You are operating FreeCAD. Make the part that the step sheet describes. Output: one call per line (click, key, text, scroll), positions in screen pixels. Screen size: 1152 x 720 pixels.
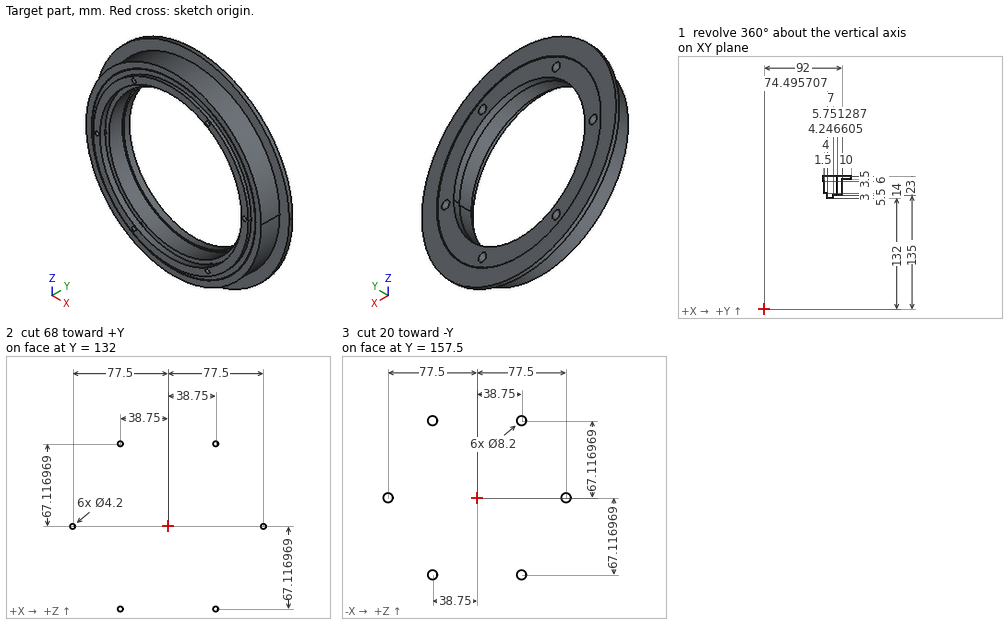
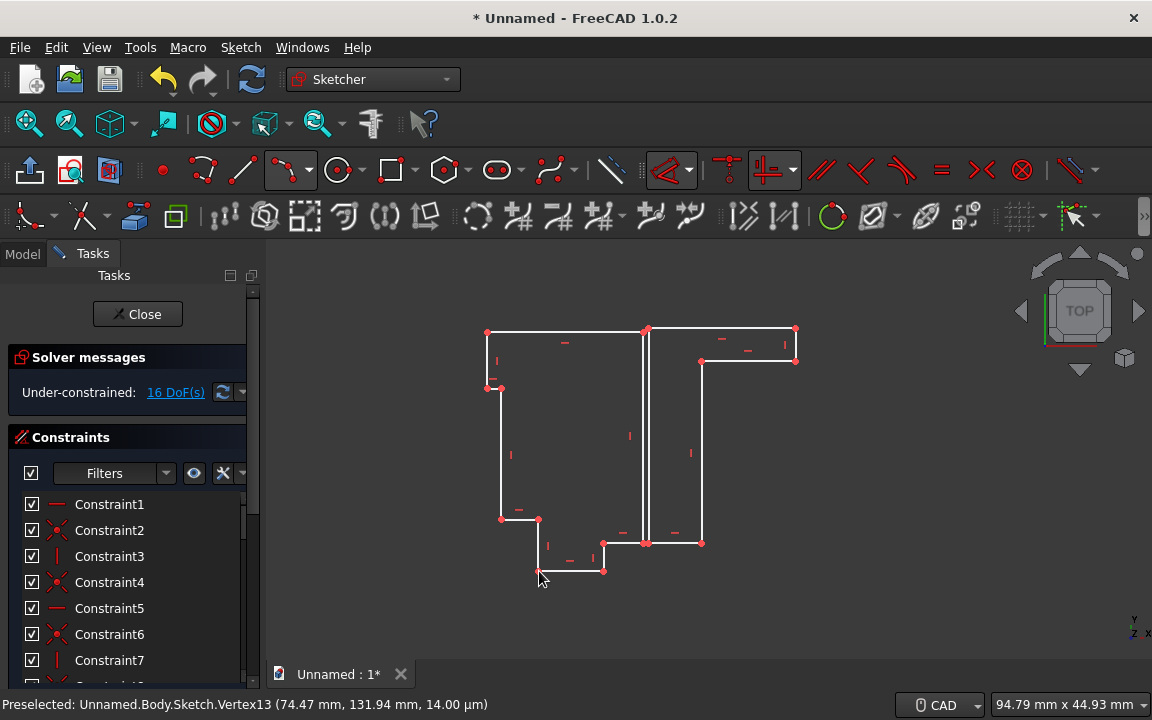
click(666, 170)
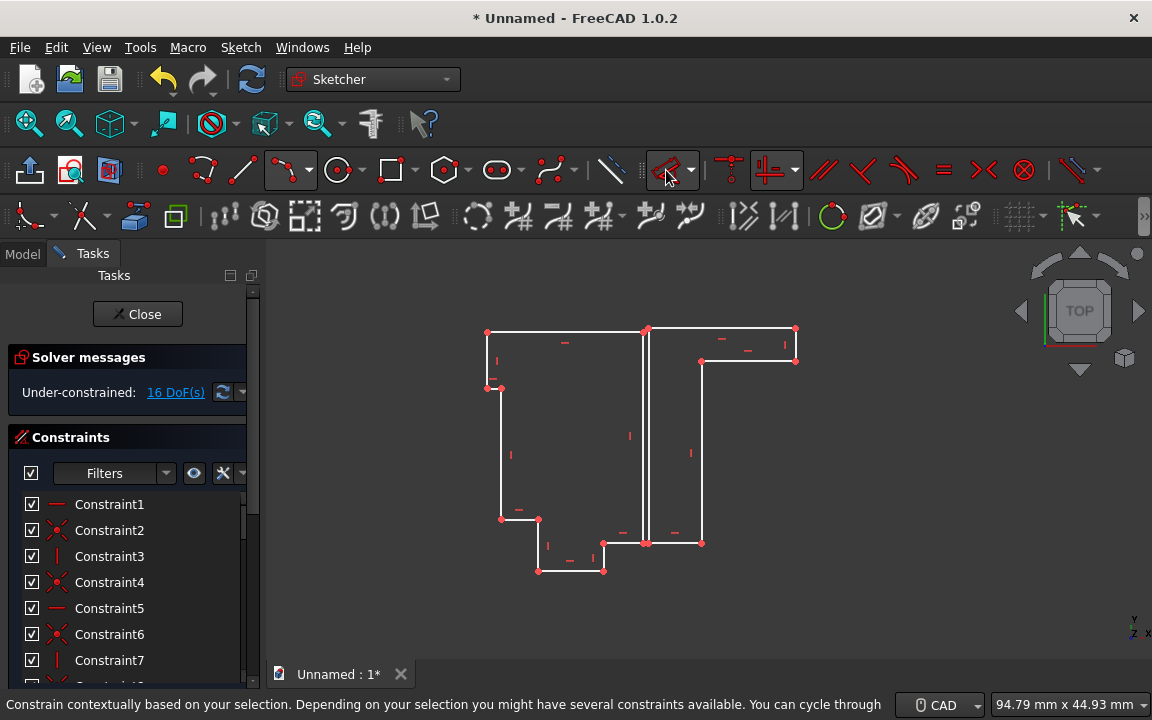
click(558, 571)
click(571, 605)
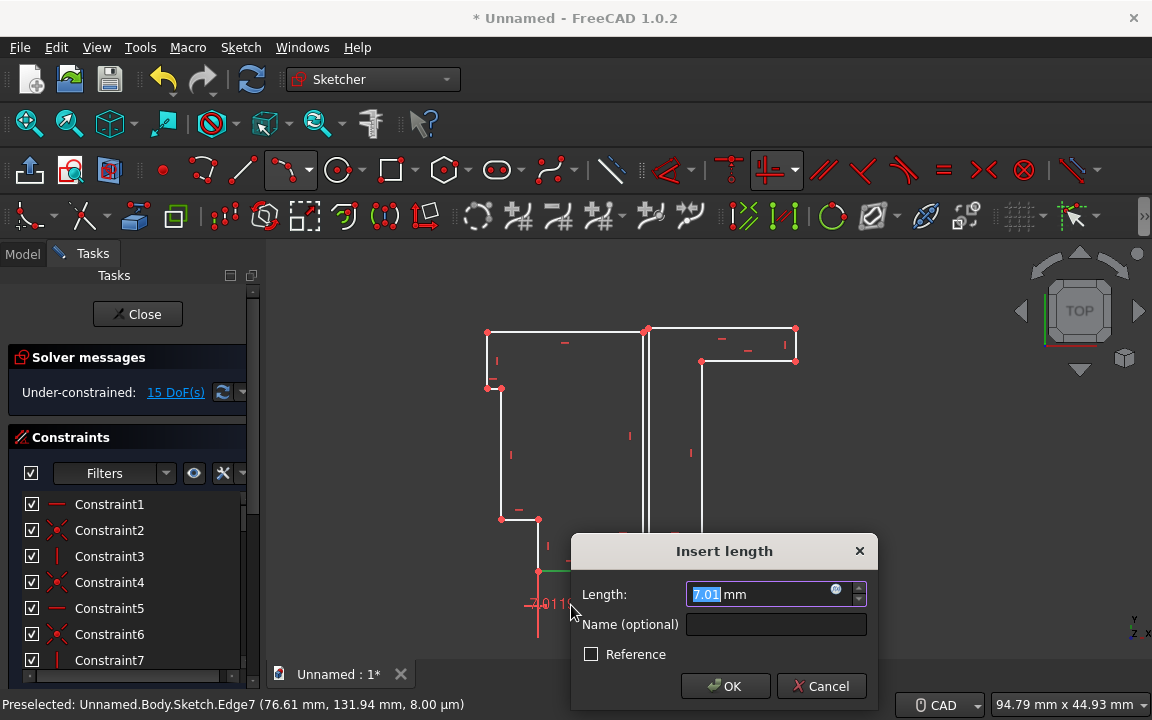
text(7)
key(Return)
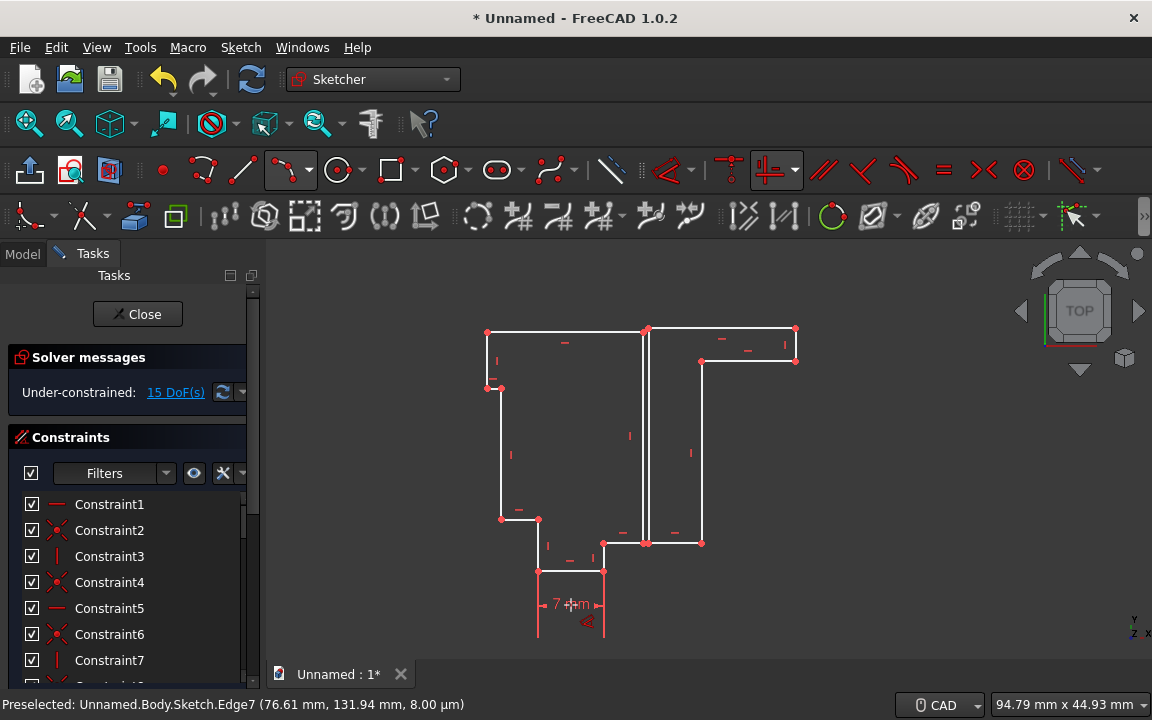
scroll(604, 560, up, 2)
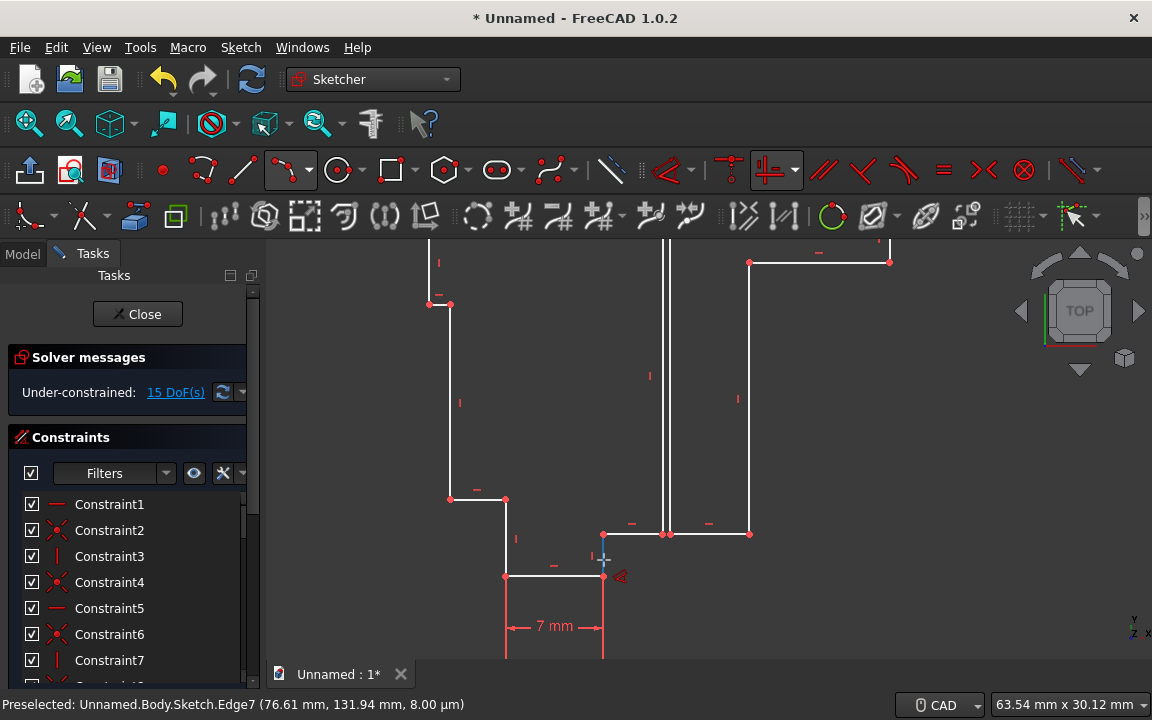
click(603, 559)
click(569, 555)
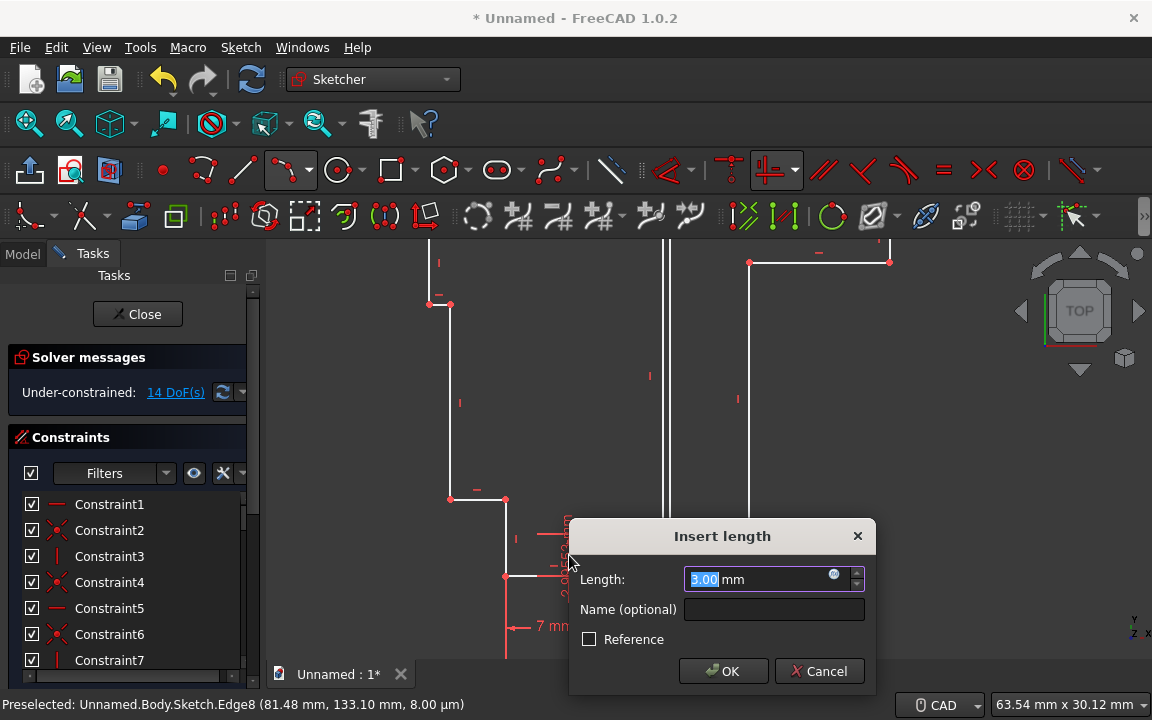
text(3)
key(Return)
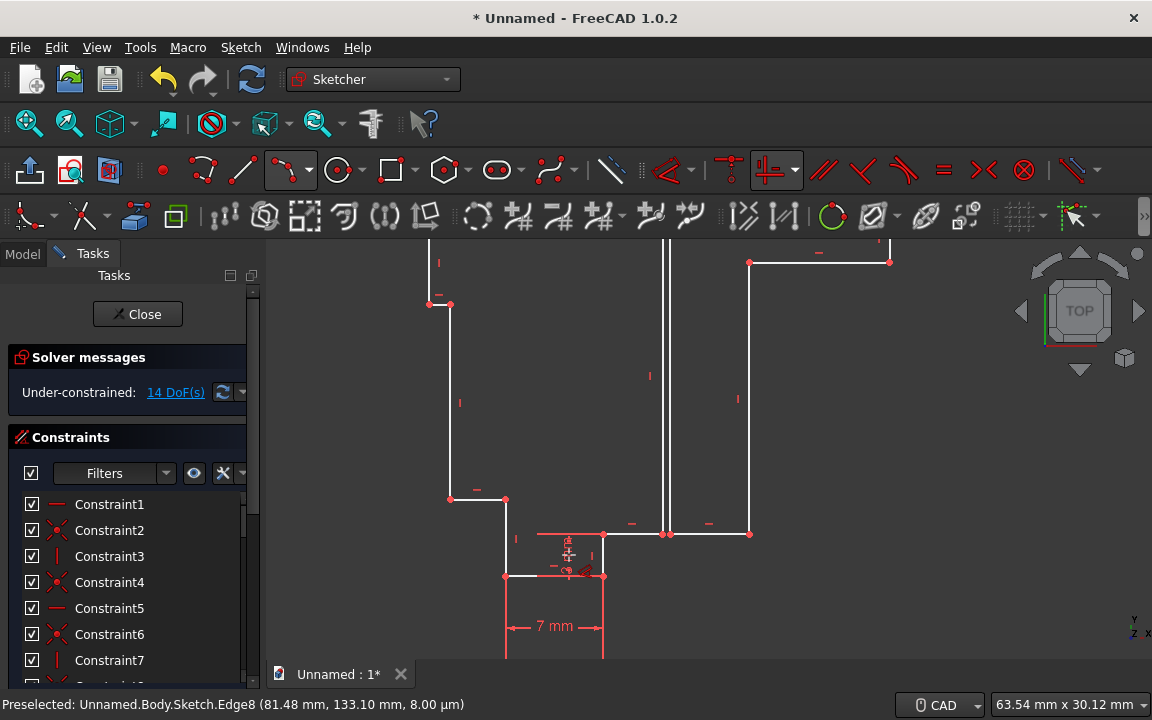
click(429, 279)
click(395, 286)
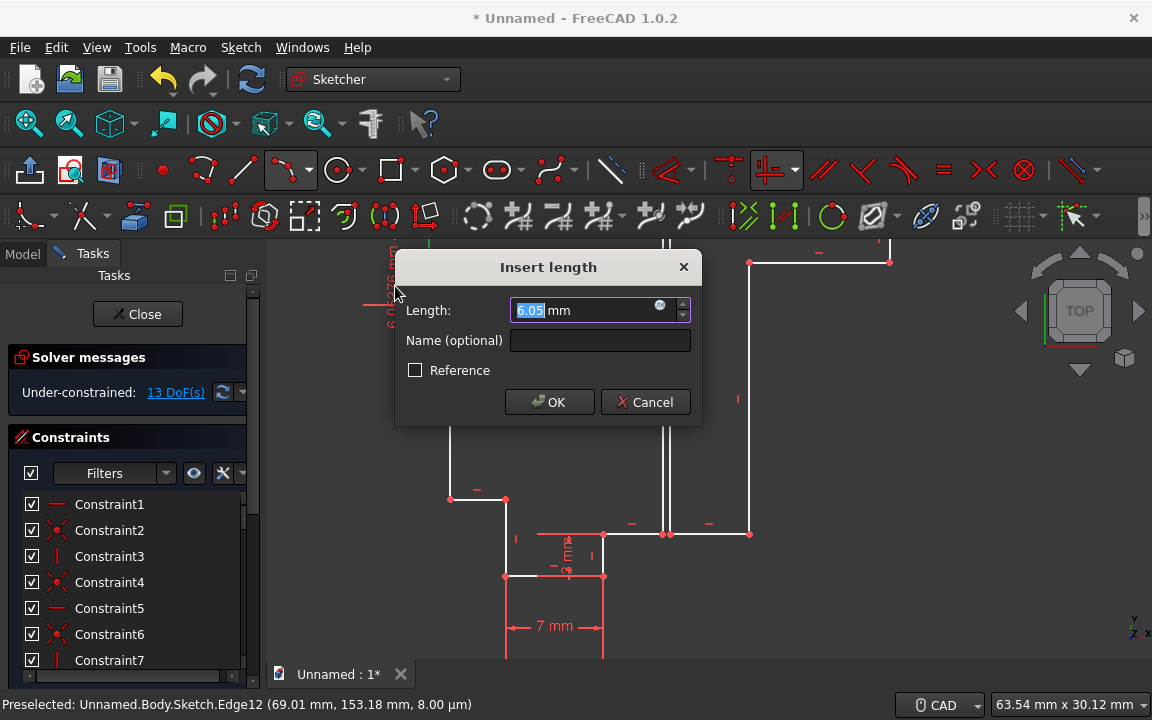
text(6)
key(Return)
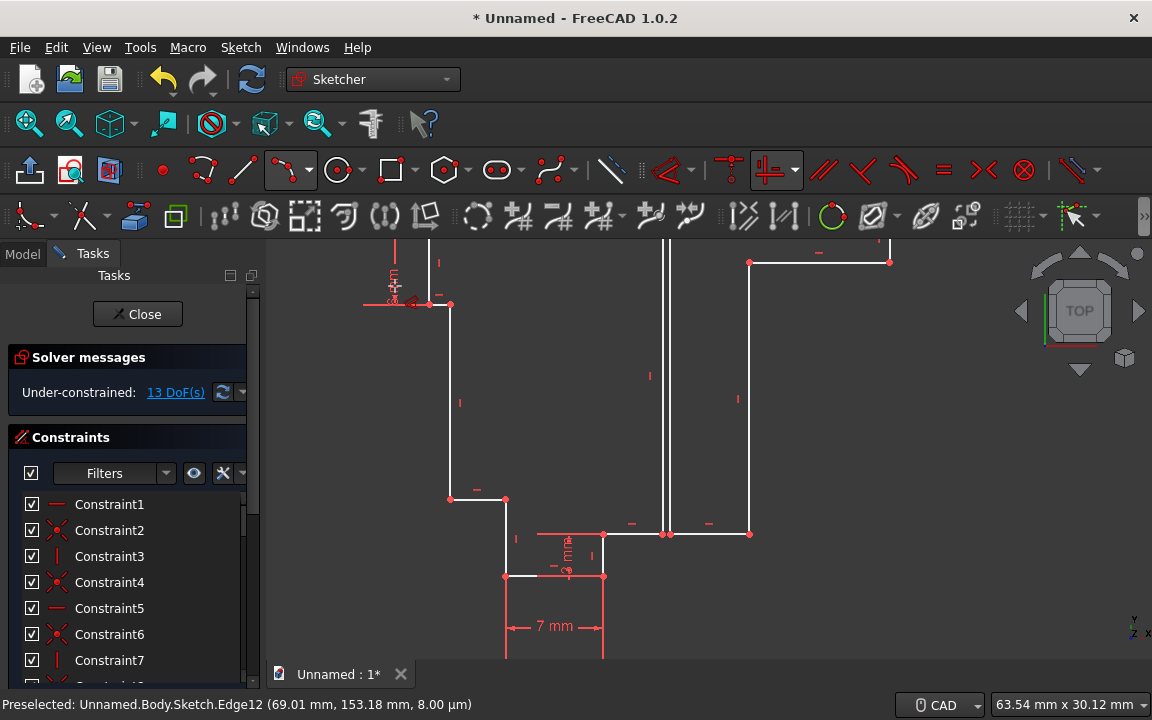
click(467, 500)
click(478, 534)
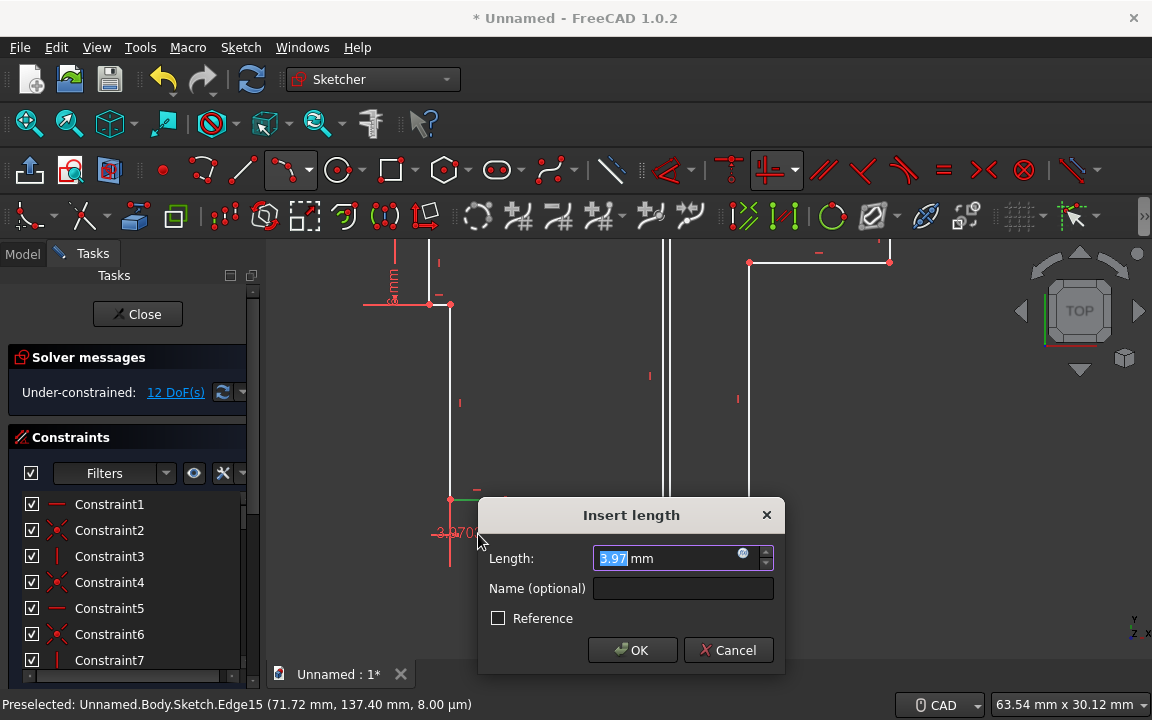
text(4)
key(Return)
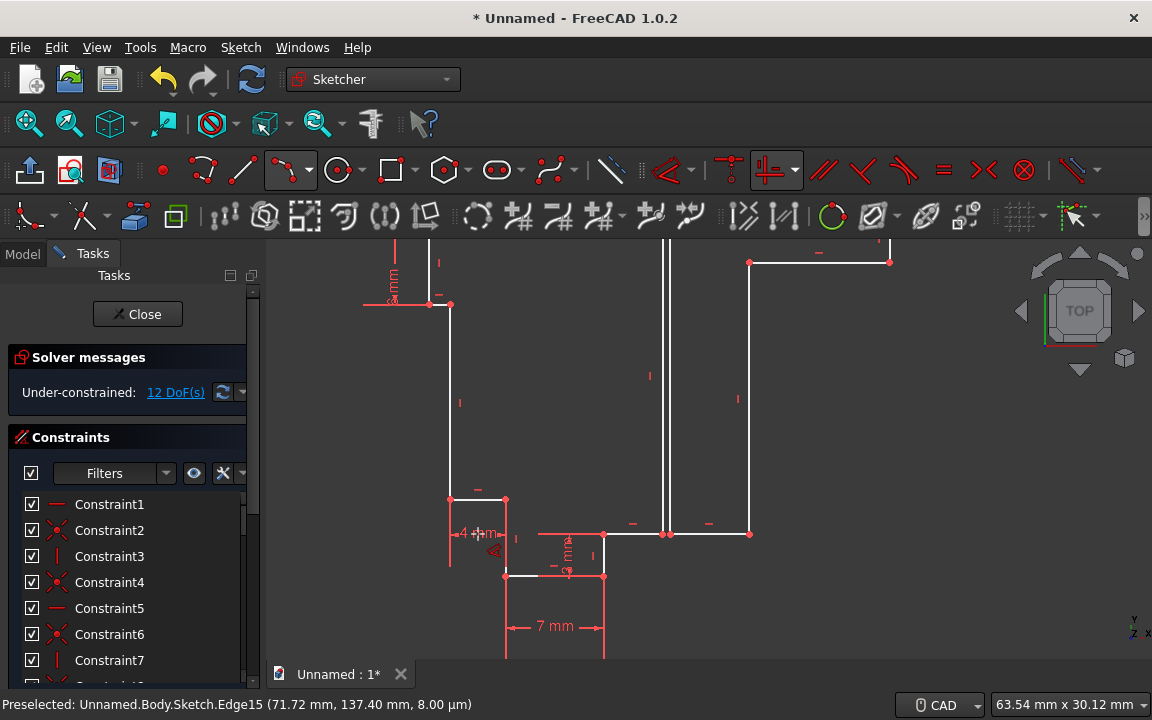
scroll(603, 561, down, 2)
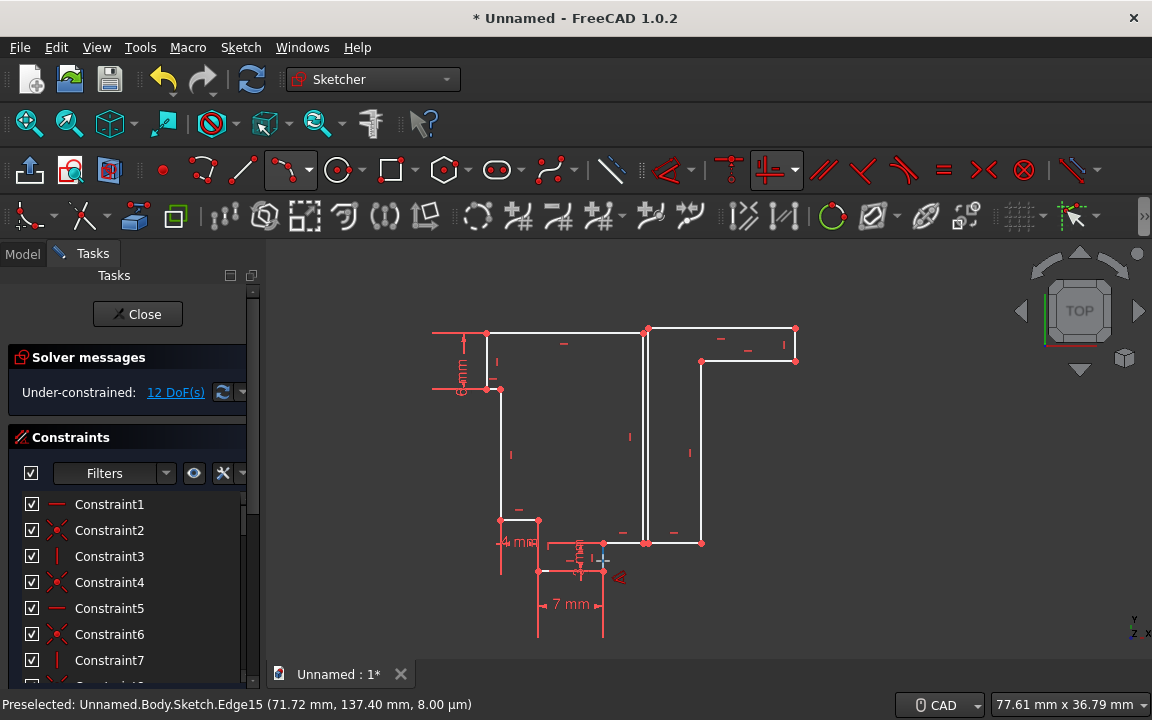
click(729, 361)
click(748, 395)